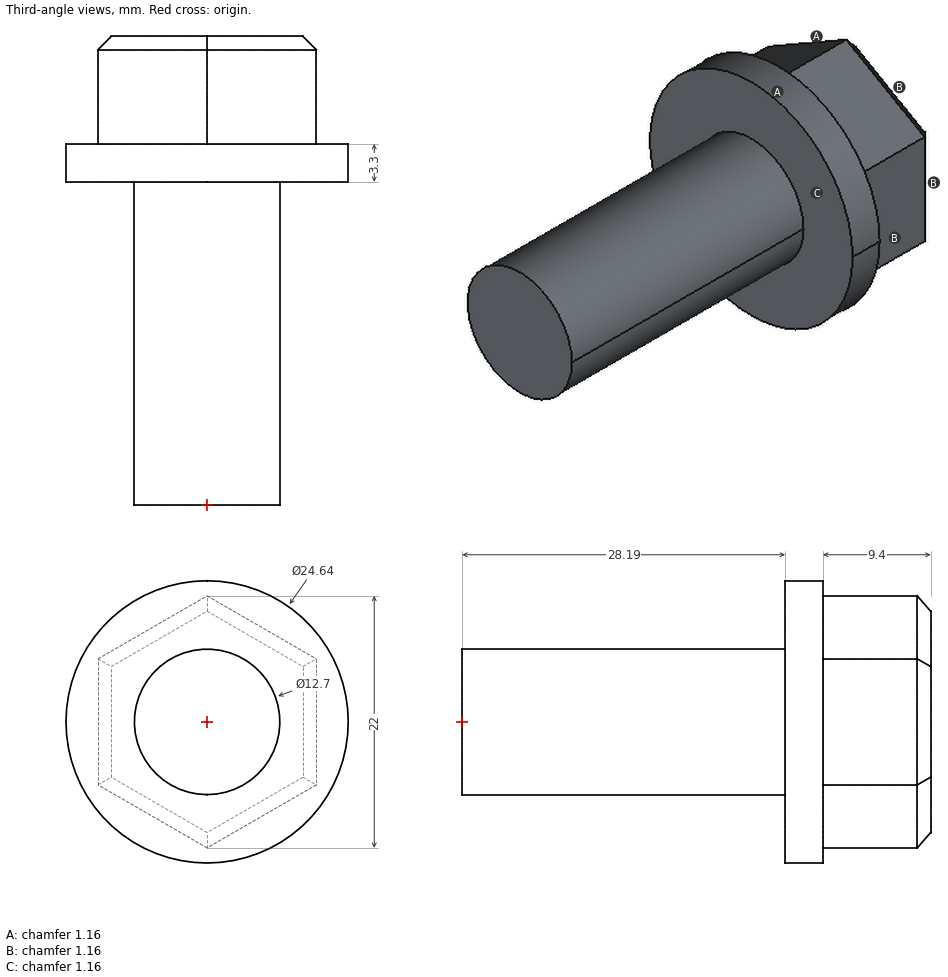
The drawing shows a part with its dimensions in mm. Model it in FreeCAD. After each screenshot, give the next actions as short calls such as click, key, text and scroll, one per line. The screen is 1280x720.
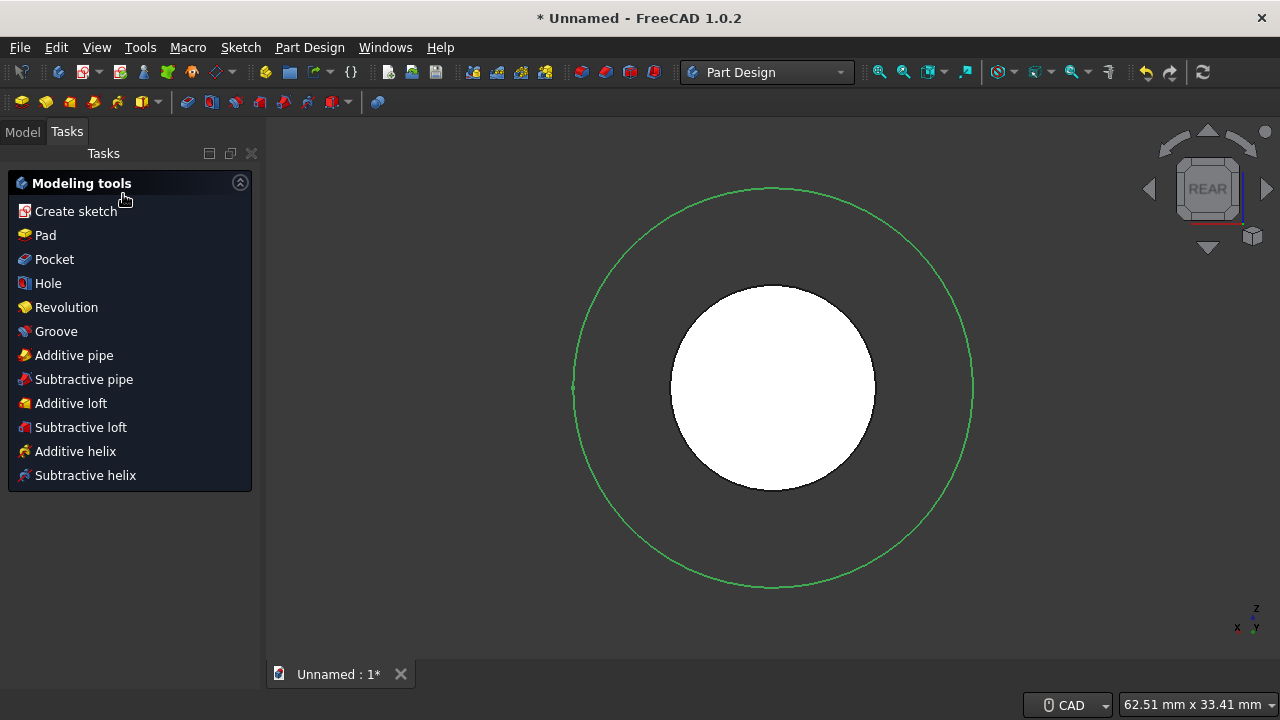
click(22, 102)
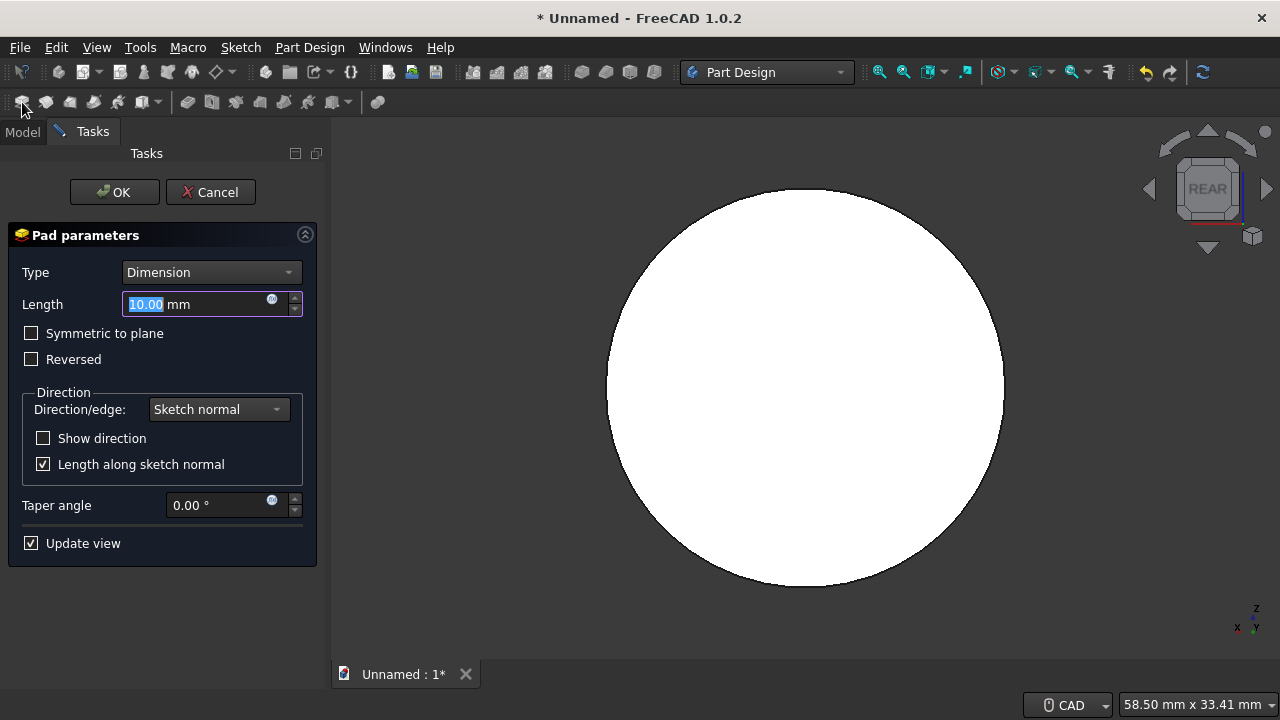
text(3.3)
key(Tab)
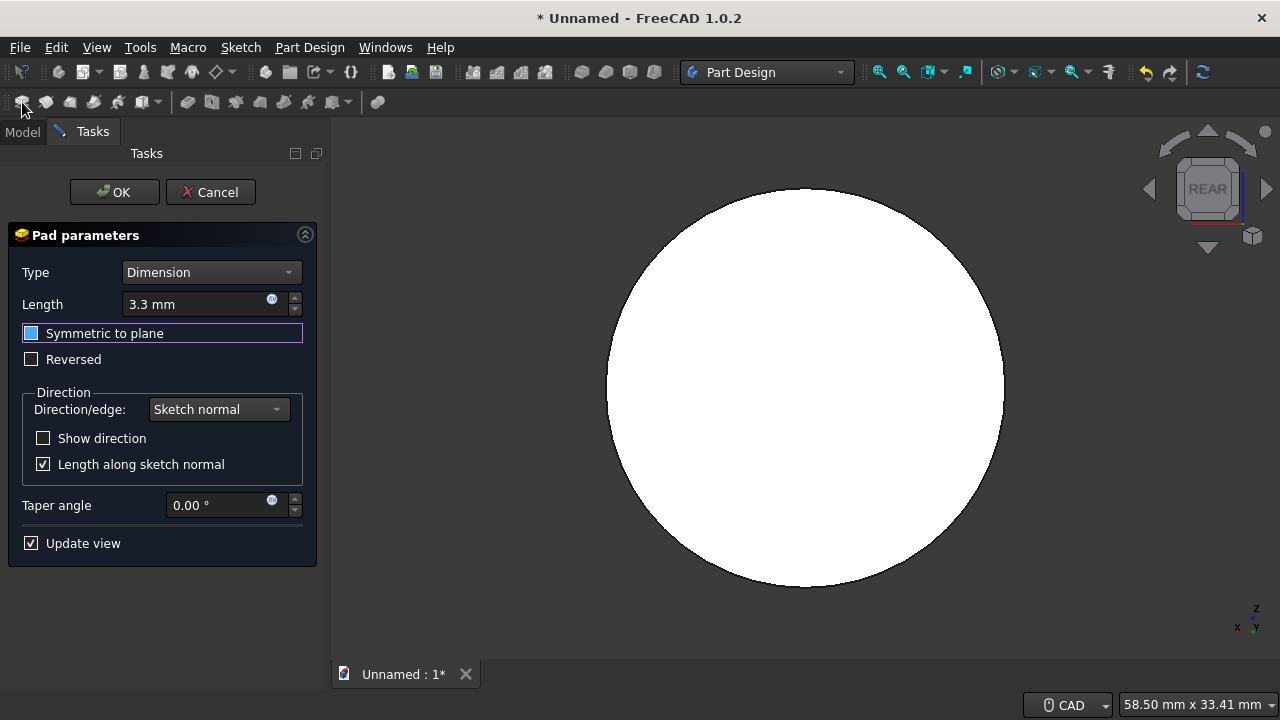
click(115, 192)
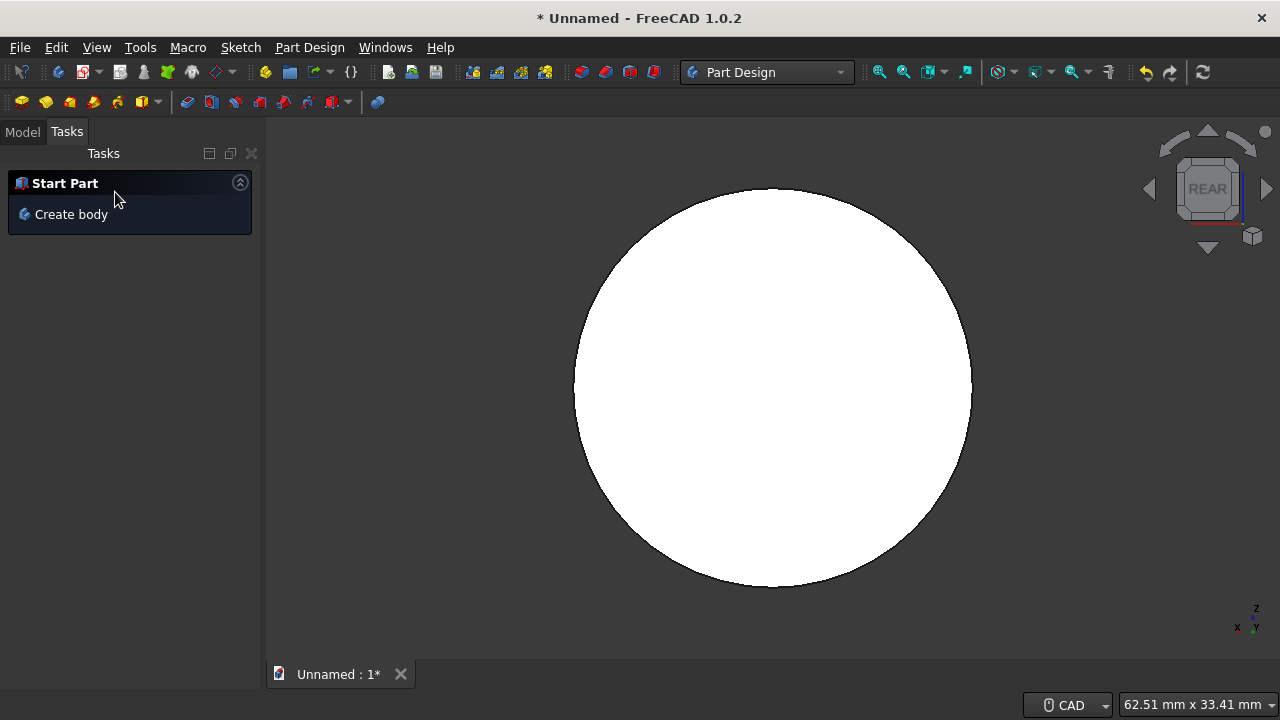
click(773, 387)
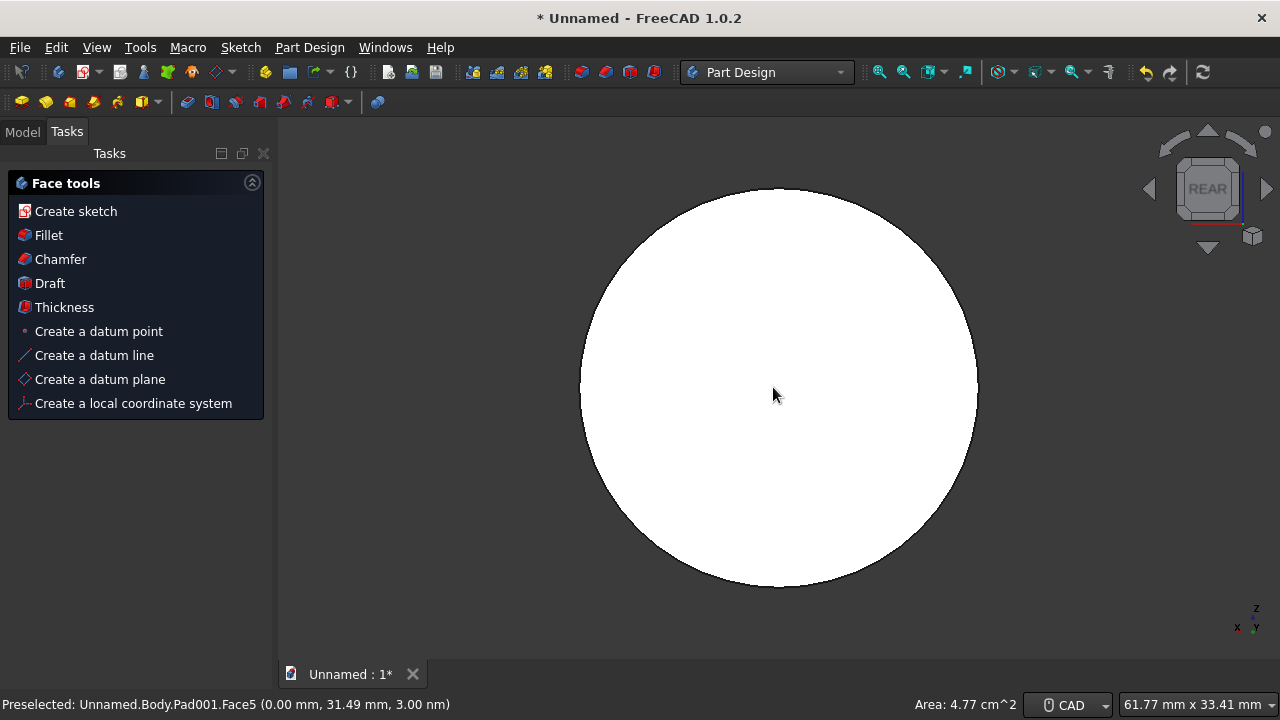
click(84, 72)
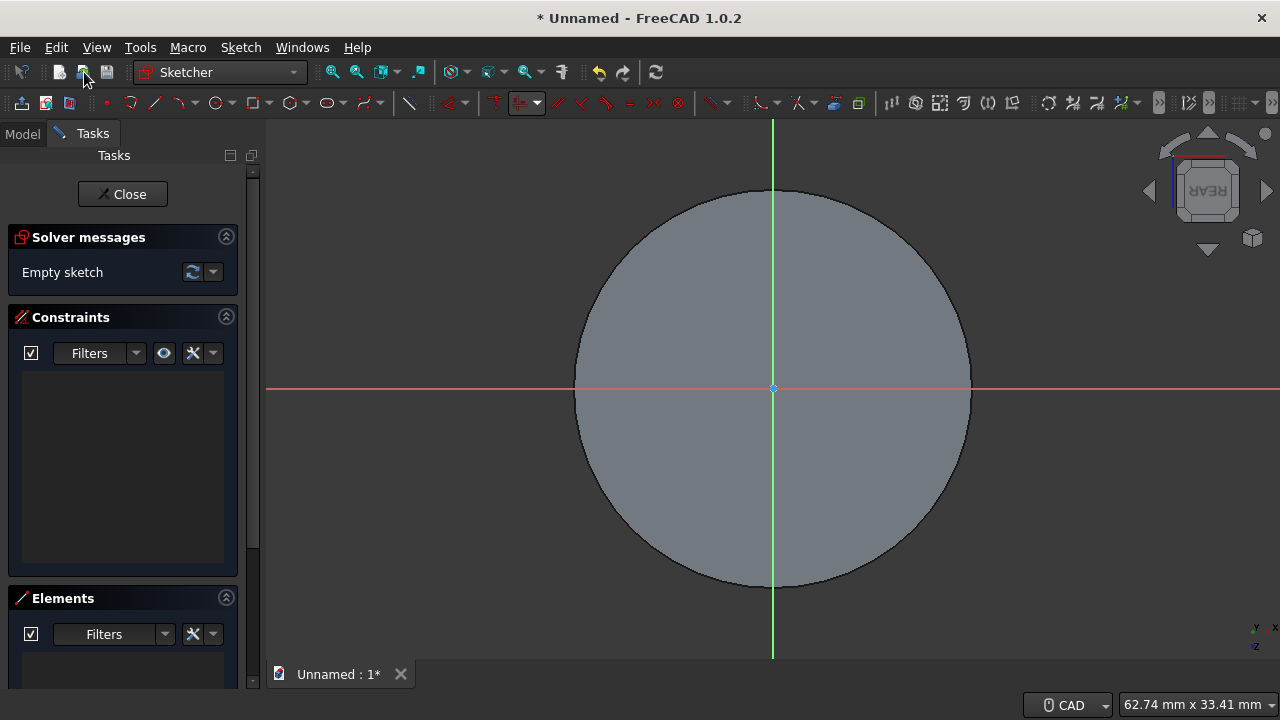
click(290, 104)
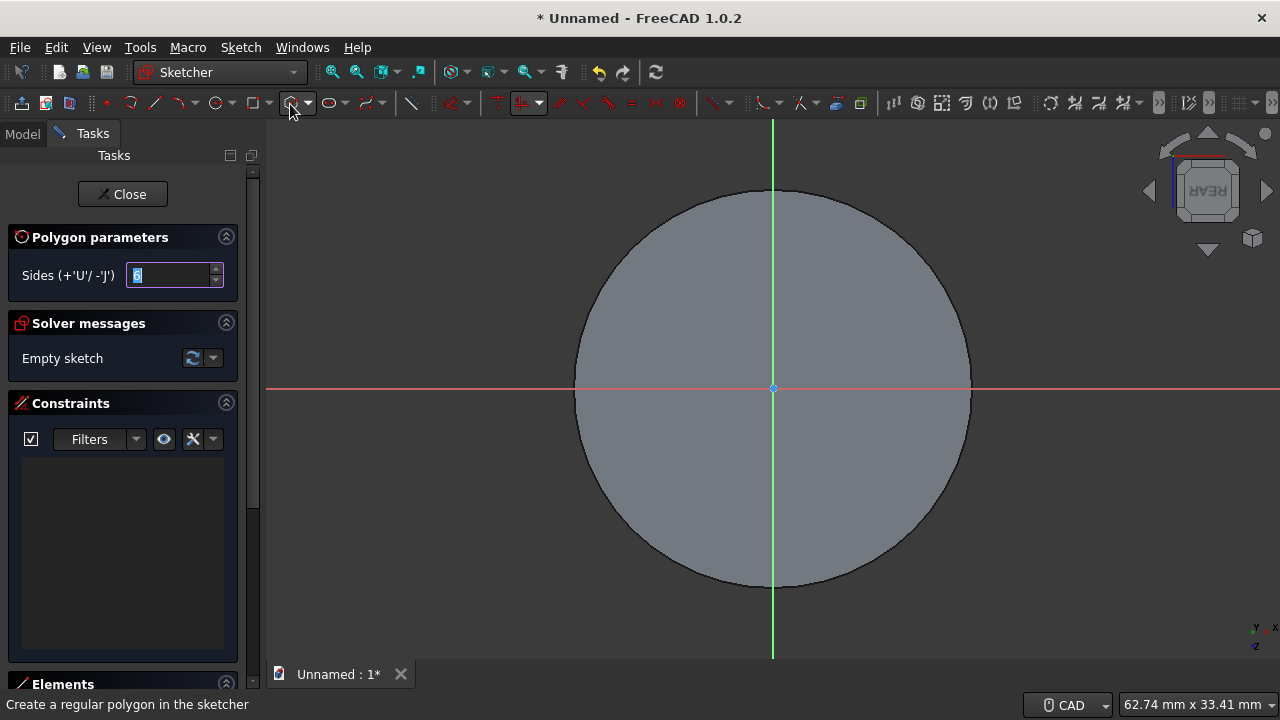
click(773, 389)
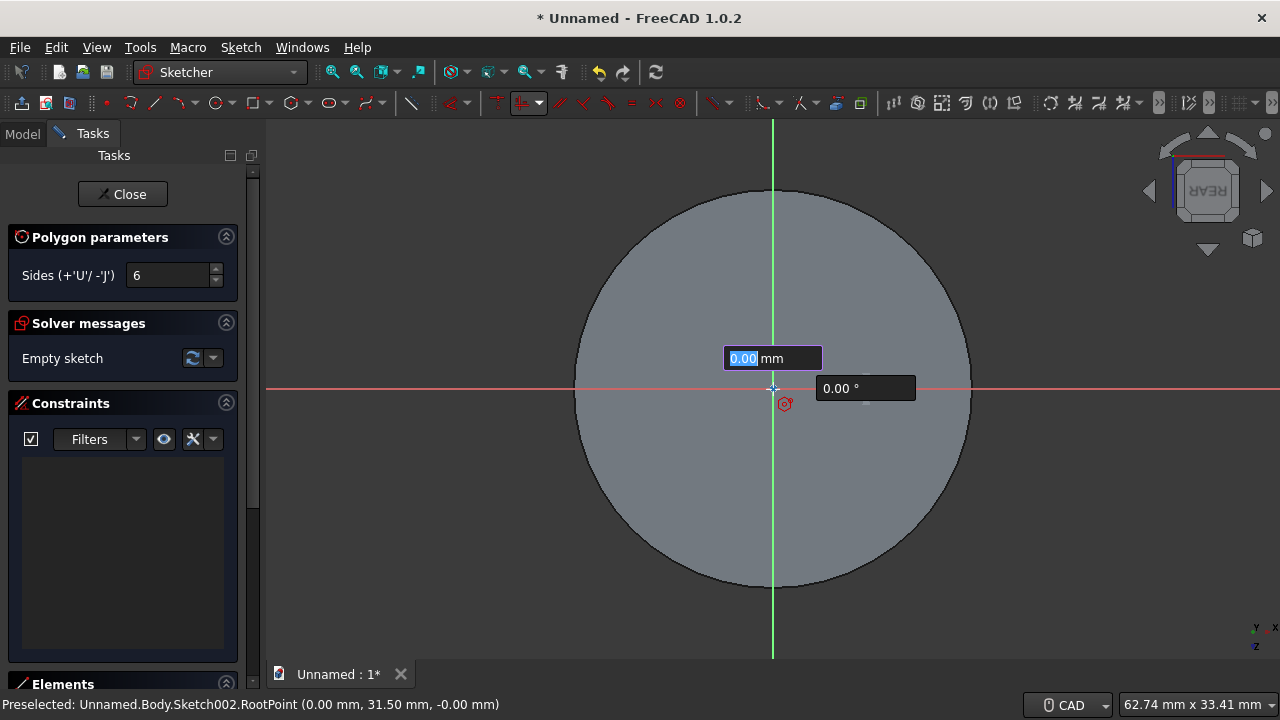
click(773, 211)
right_click(773, 211)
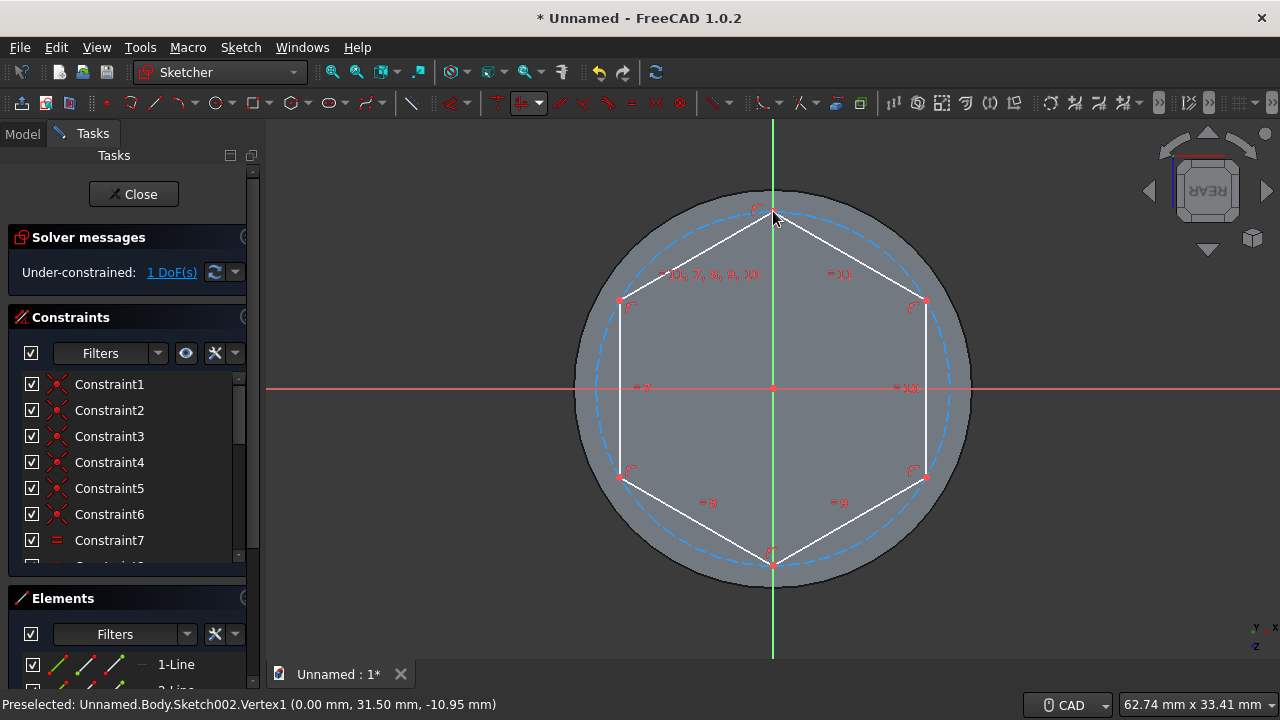
click(773, 566)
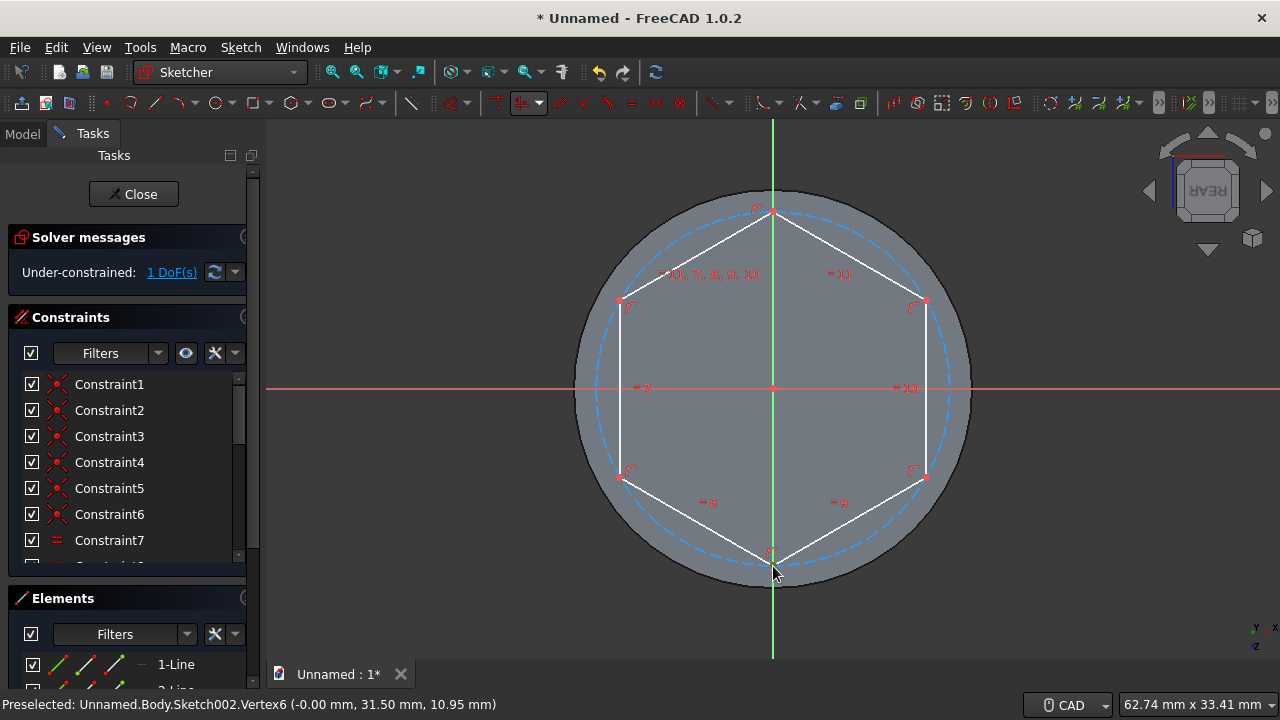
click(773, 212)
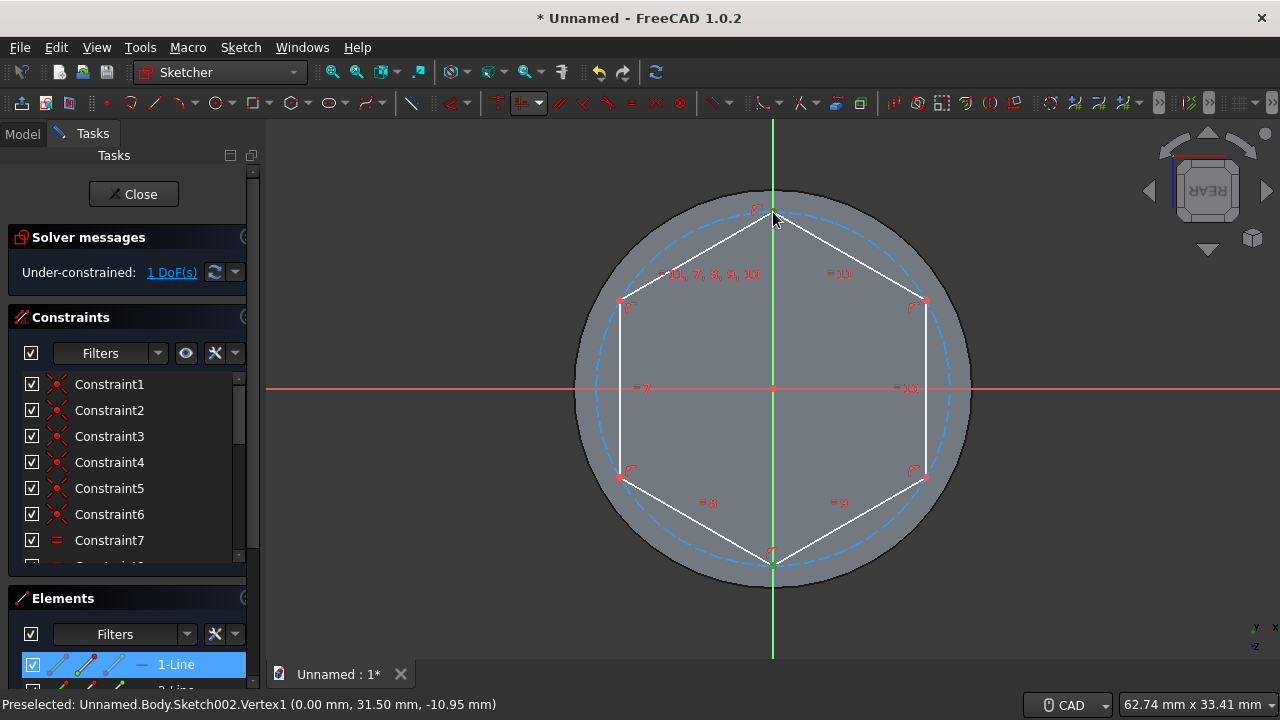
click(470, 104)